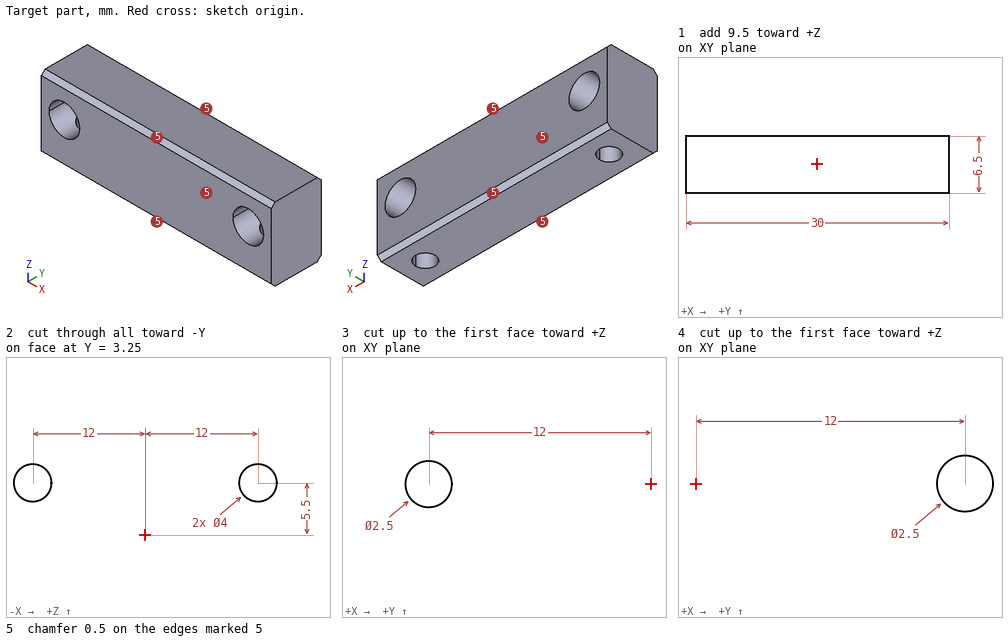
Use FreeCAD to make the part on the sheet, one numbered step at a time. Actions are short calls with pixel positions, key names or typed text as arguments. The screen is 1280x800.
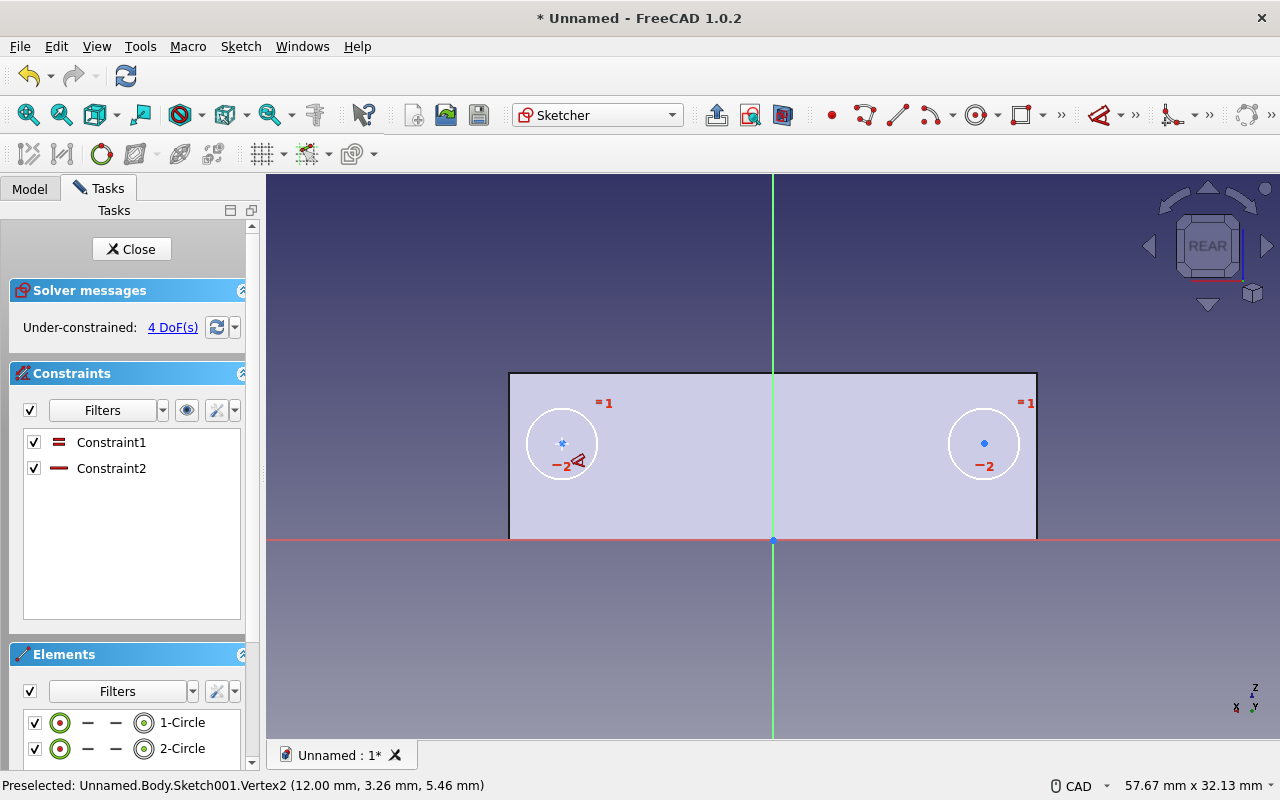
click(1009, 419)
click(1032, 396)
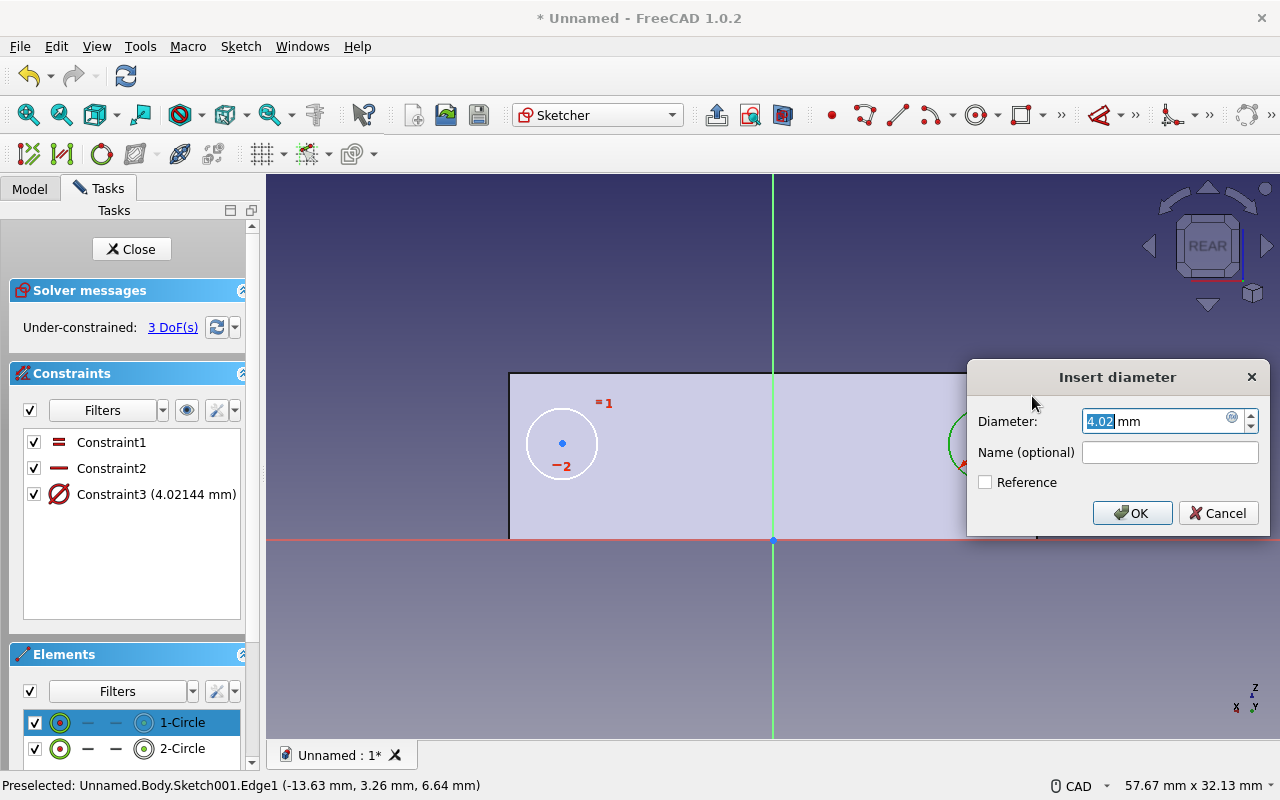
text(4)
key(Return)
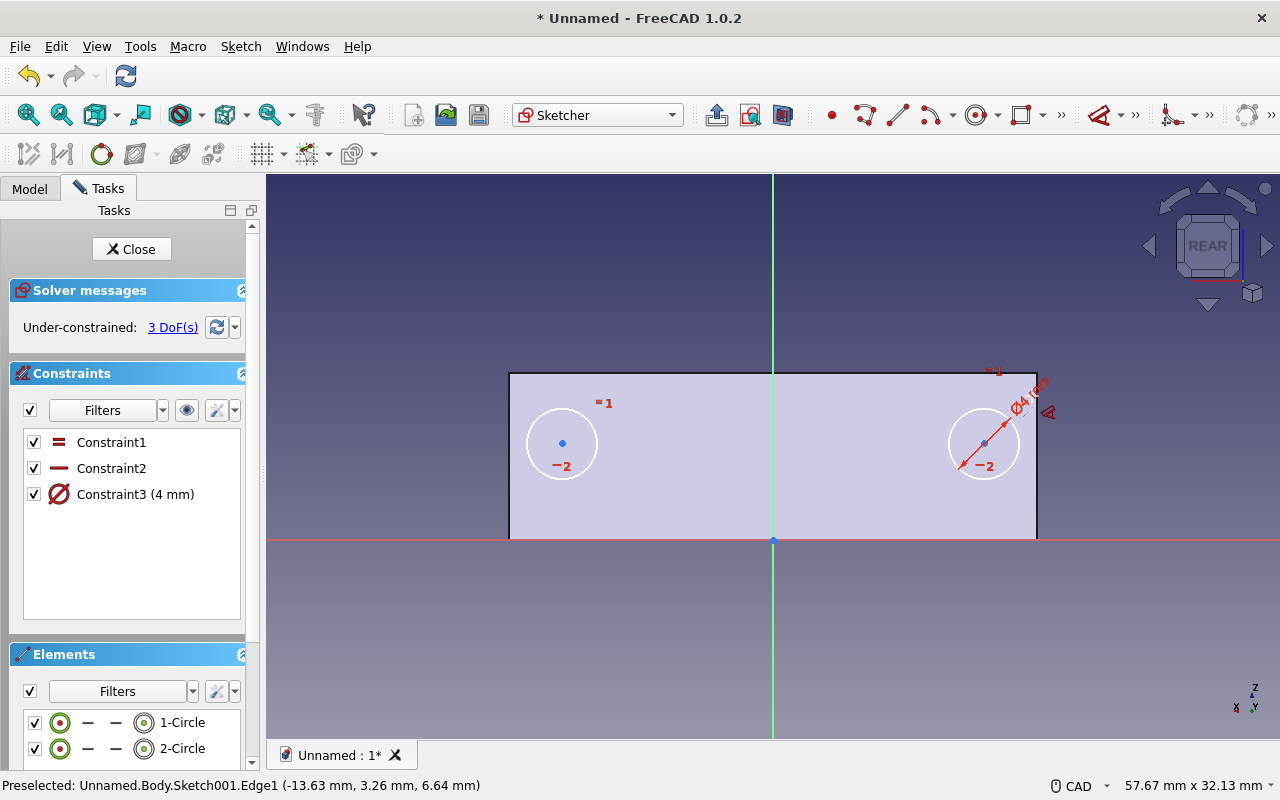
click(984, 444)
click(879, 574)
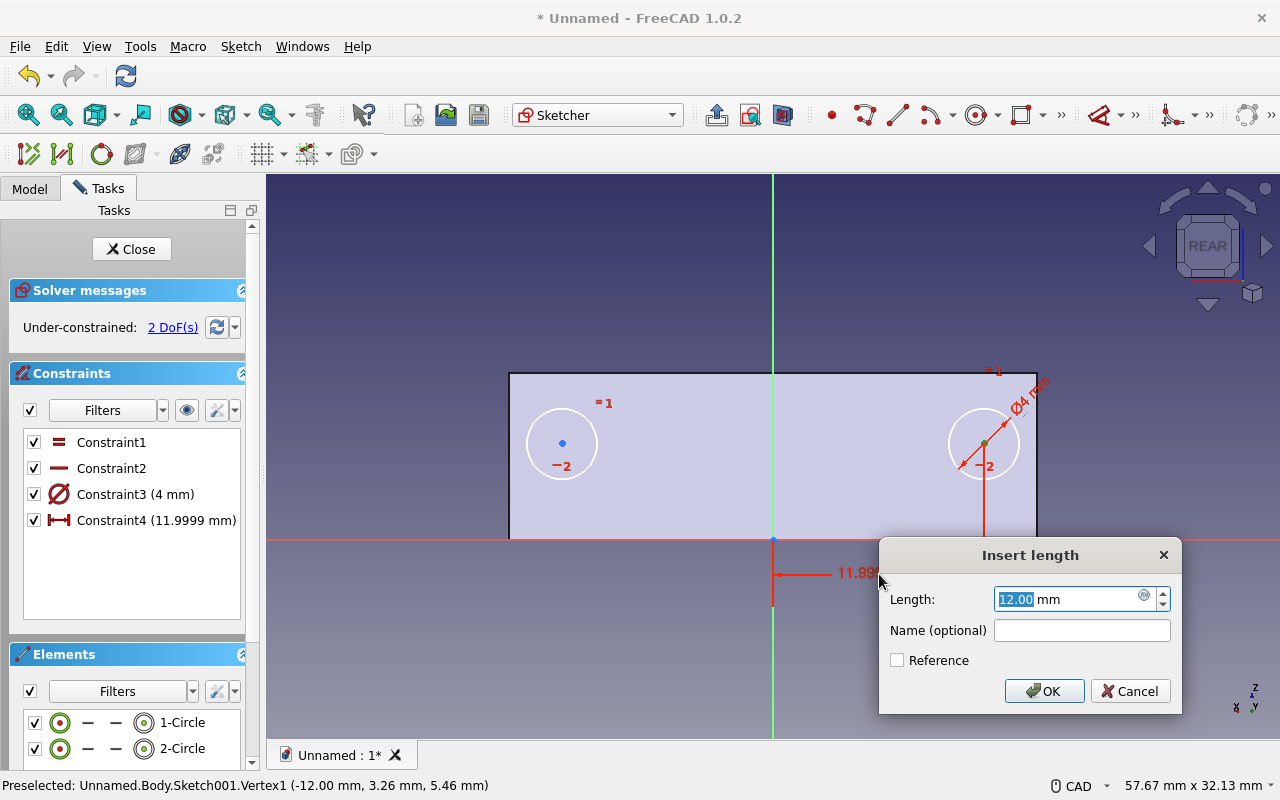
text(12)
key(Return)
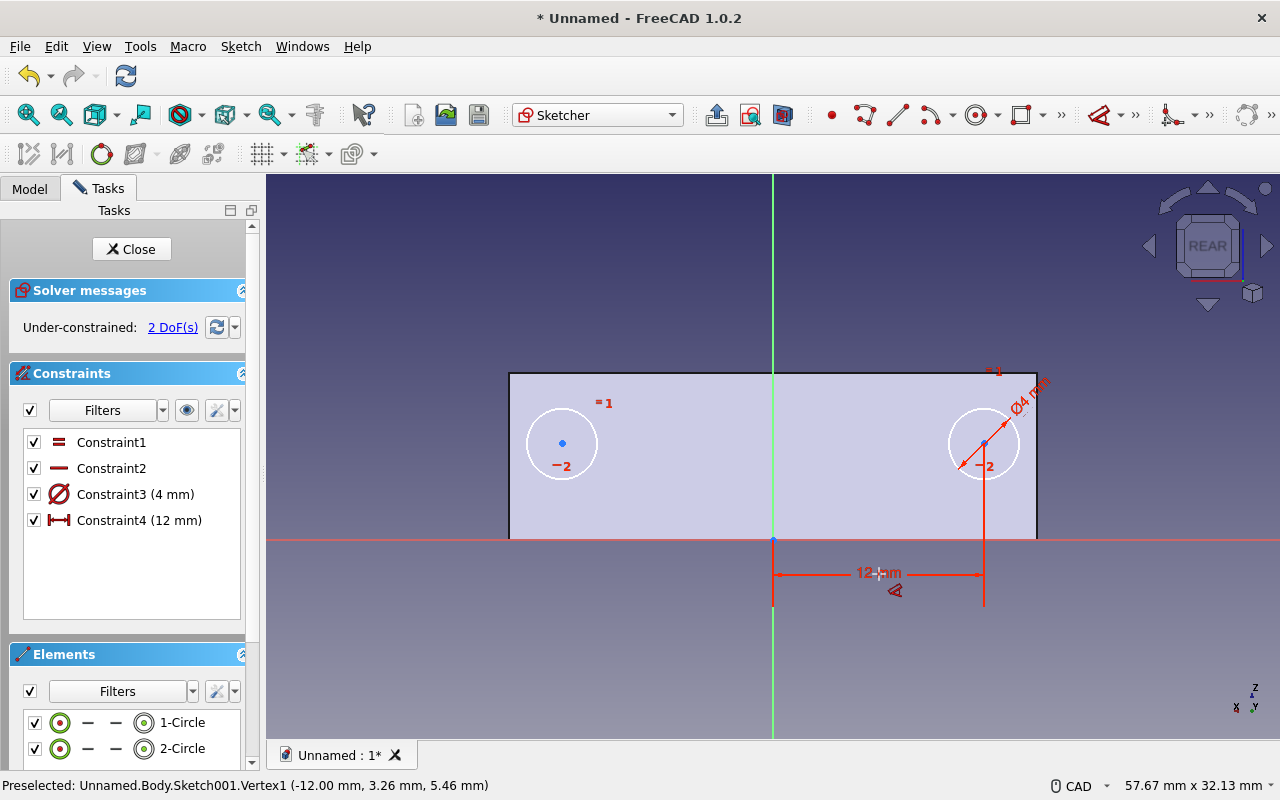
click(562, 444)
click(667, 574)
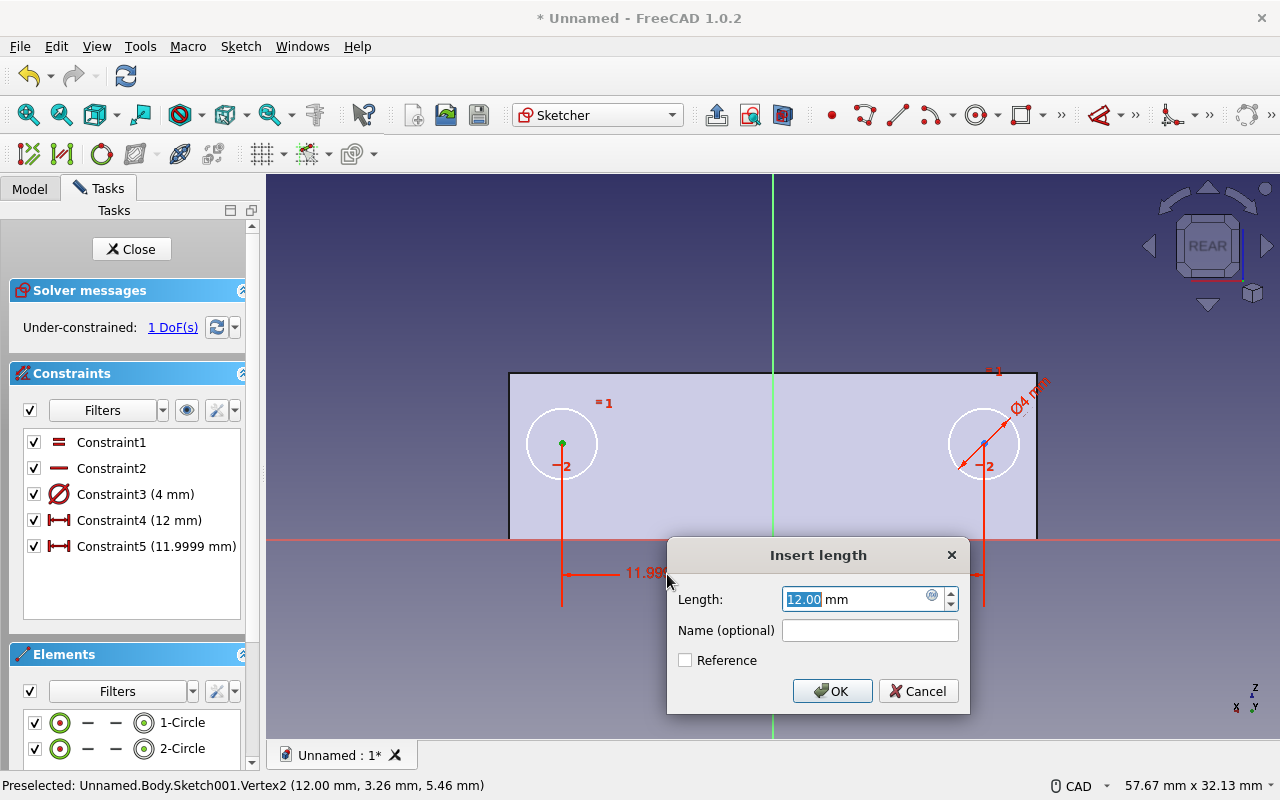
text(12)
key(Return)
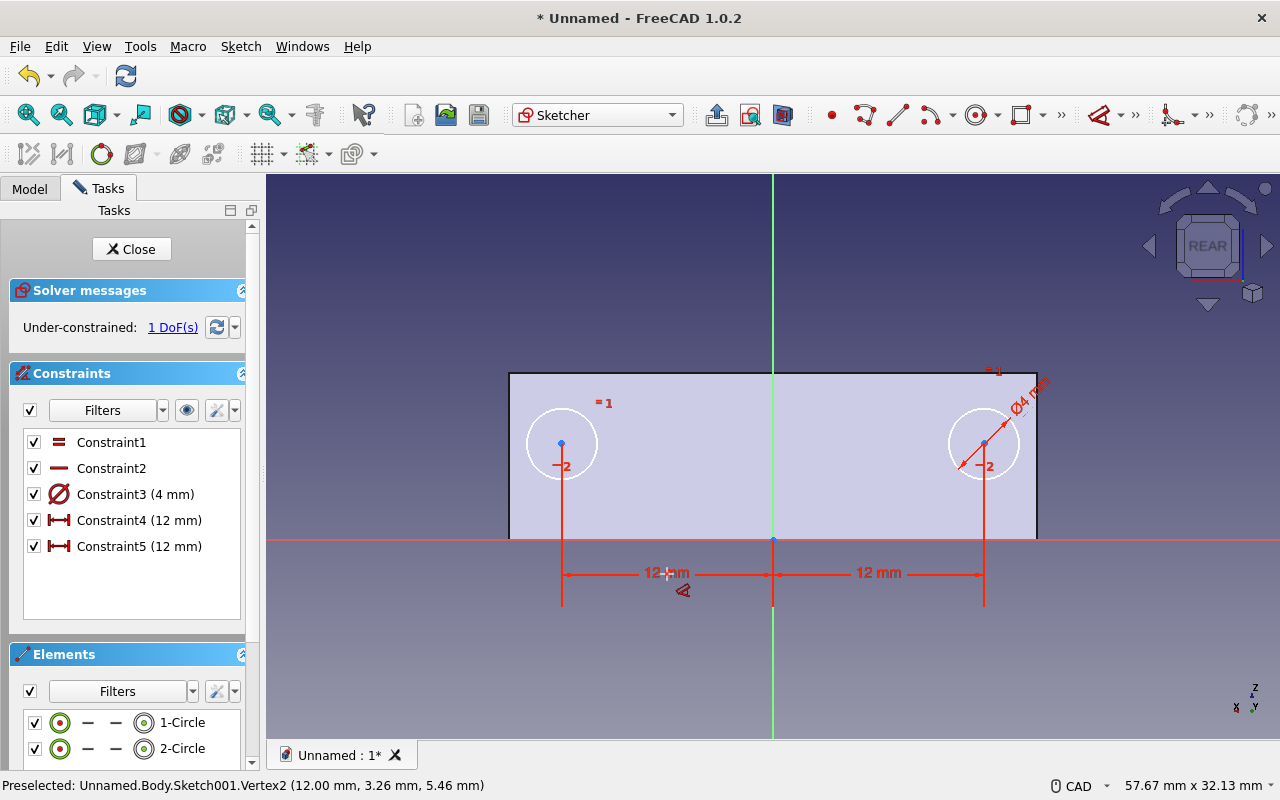
click(984, 444)
click(1018, 492)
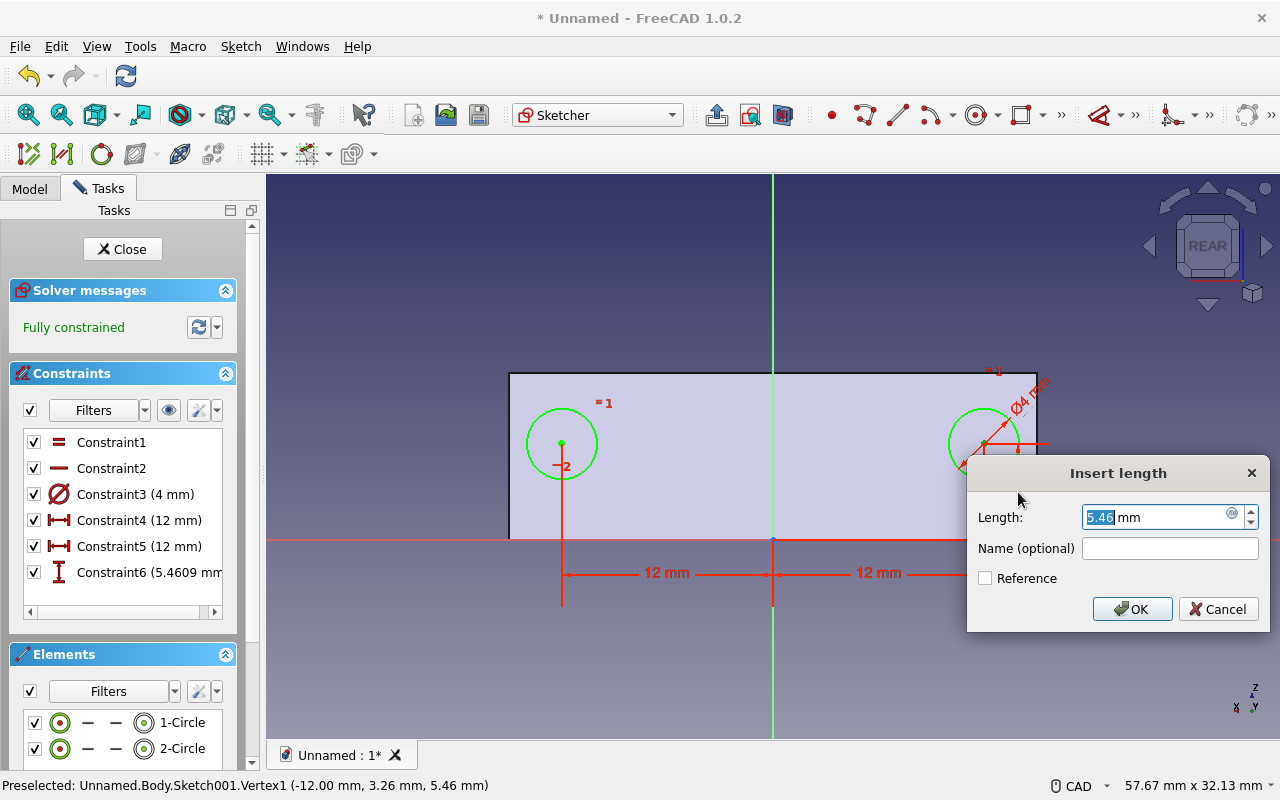
text(5.5)
key(Return)
key(Escape)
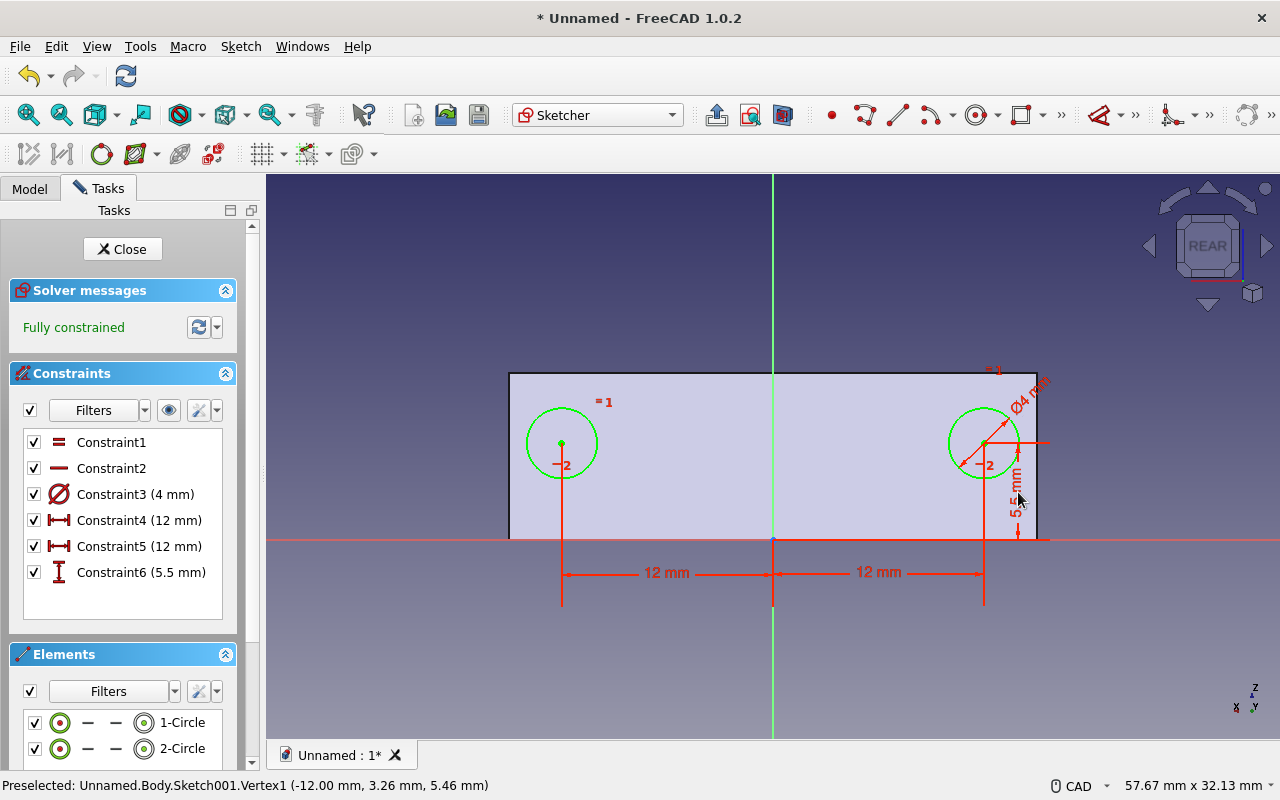
click(123, 249)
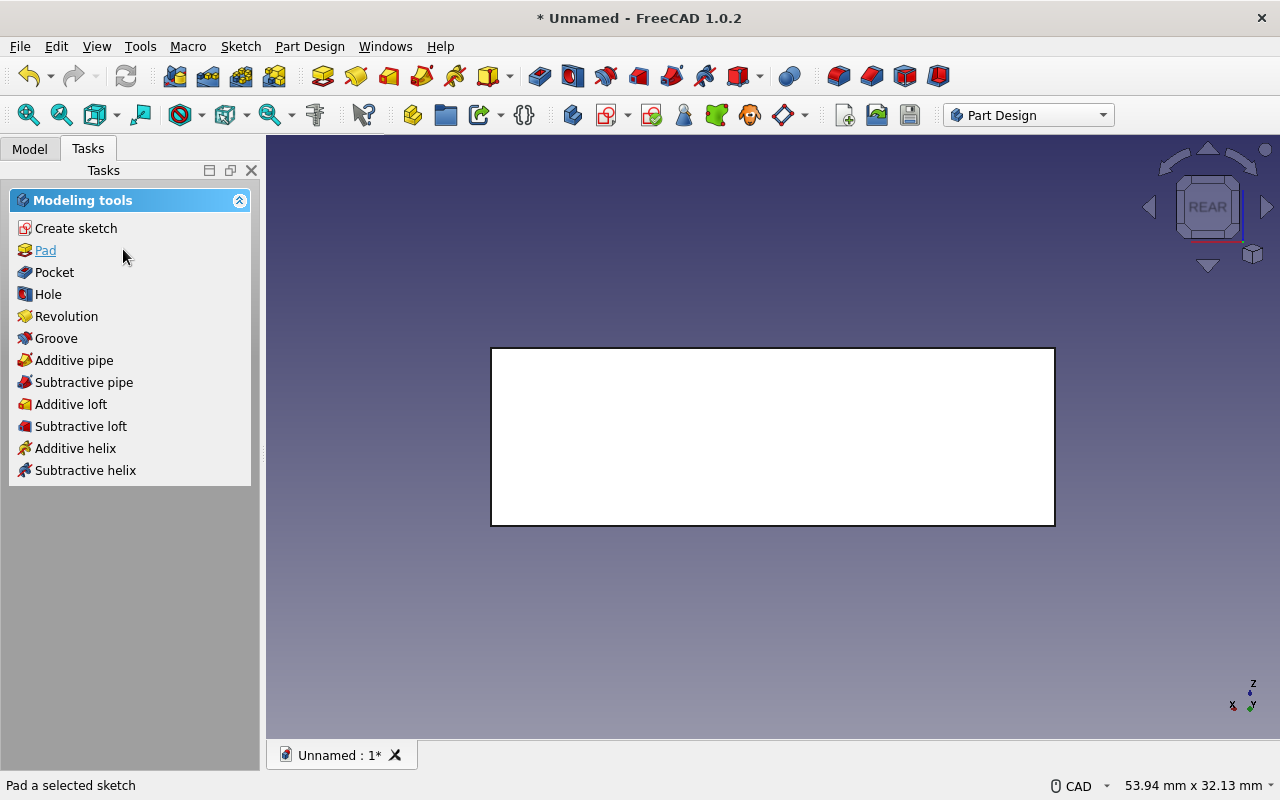
click(540, 76)